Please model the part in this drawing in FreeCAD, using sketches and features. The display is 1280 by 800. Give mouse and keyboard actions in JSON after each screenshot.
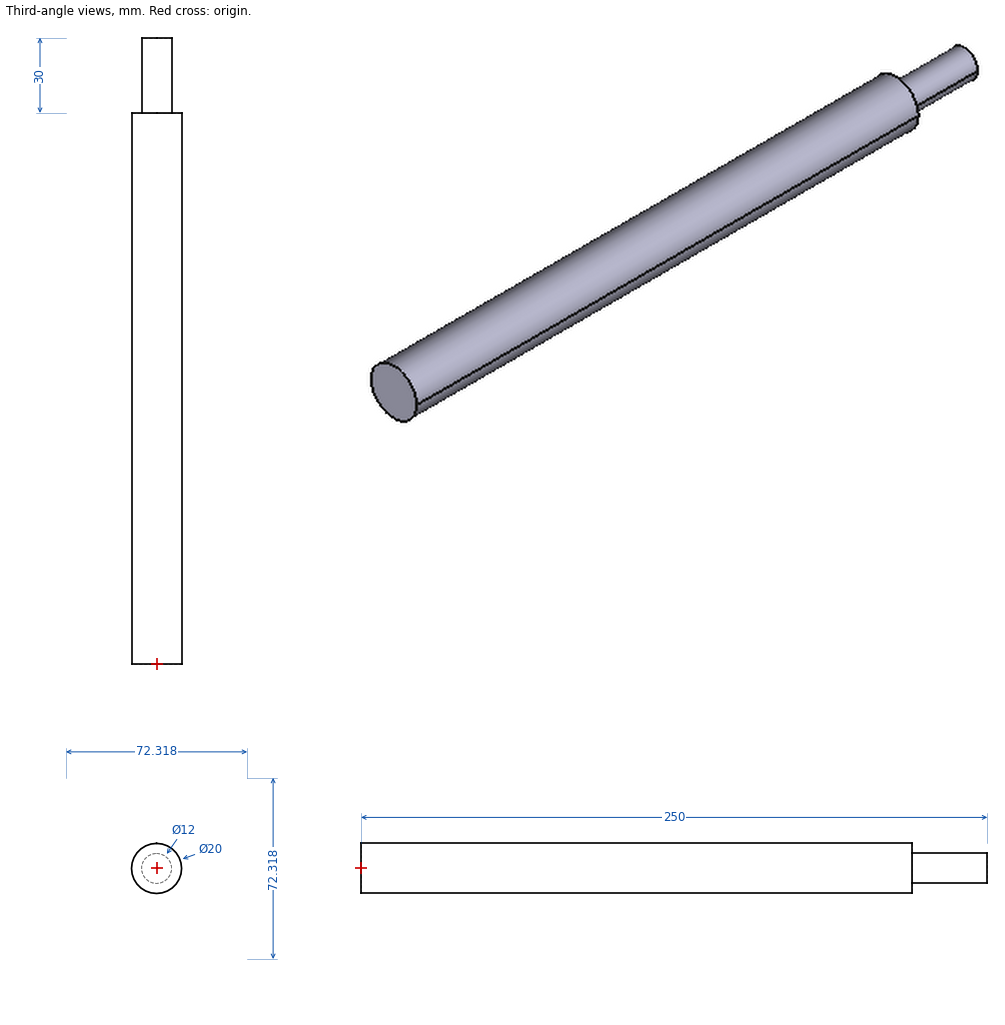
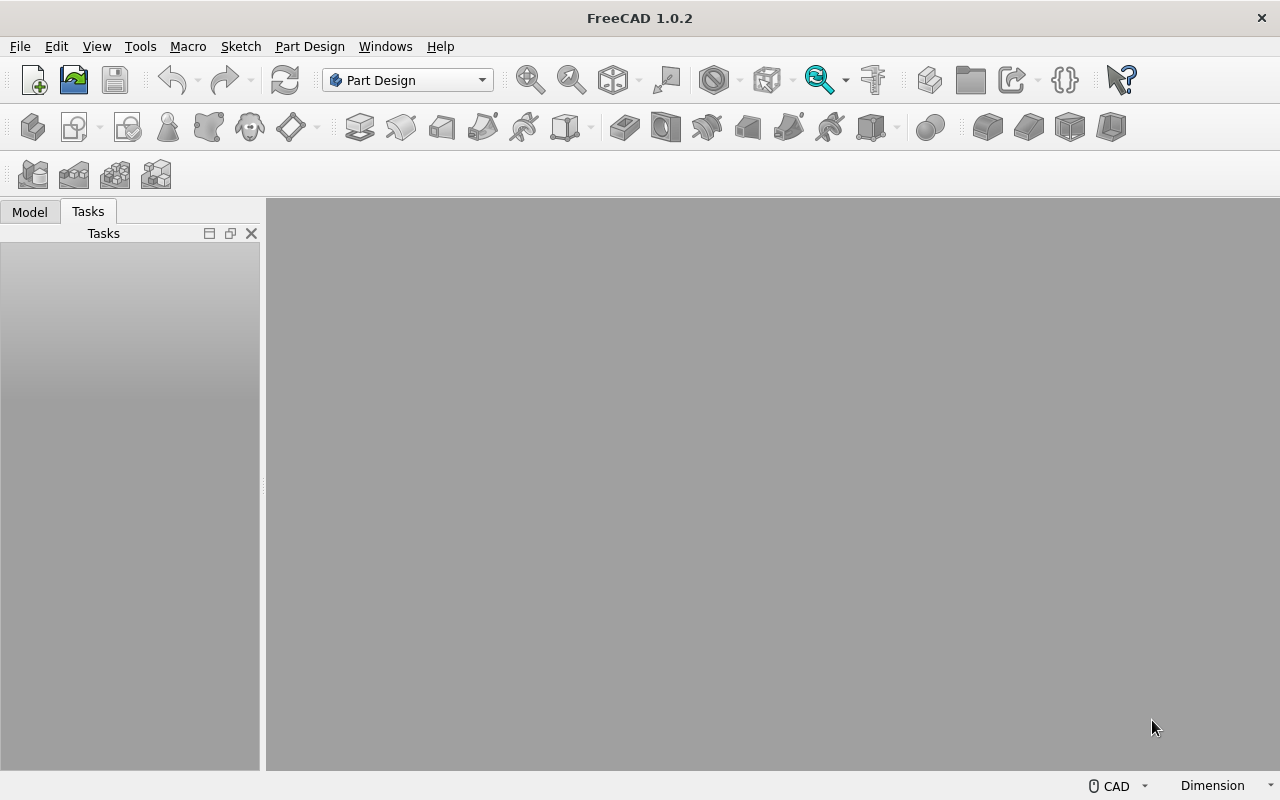
{"action": "left_click", "coordinate": [33, 80]}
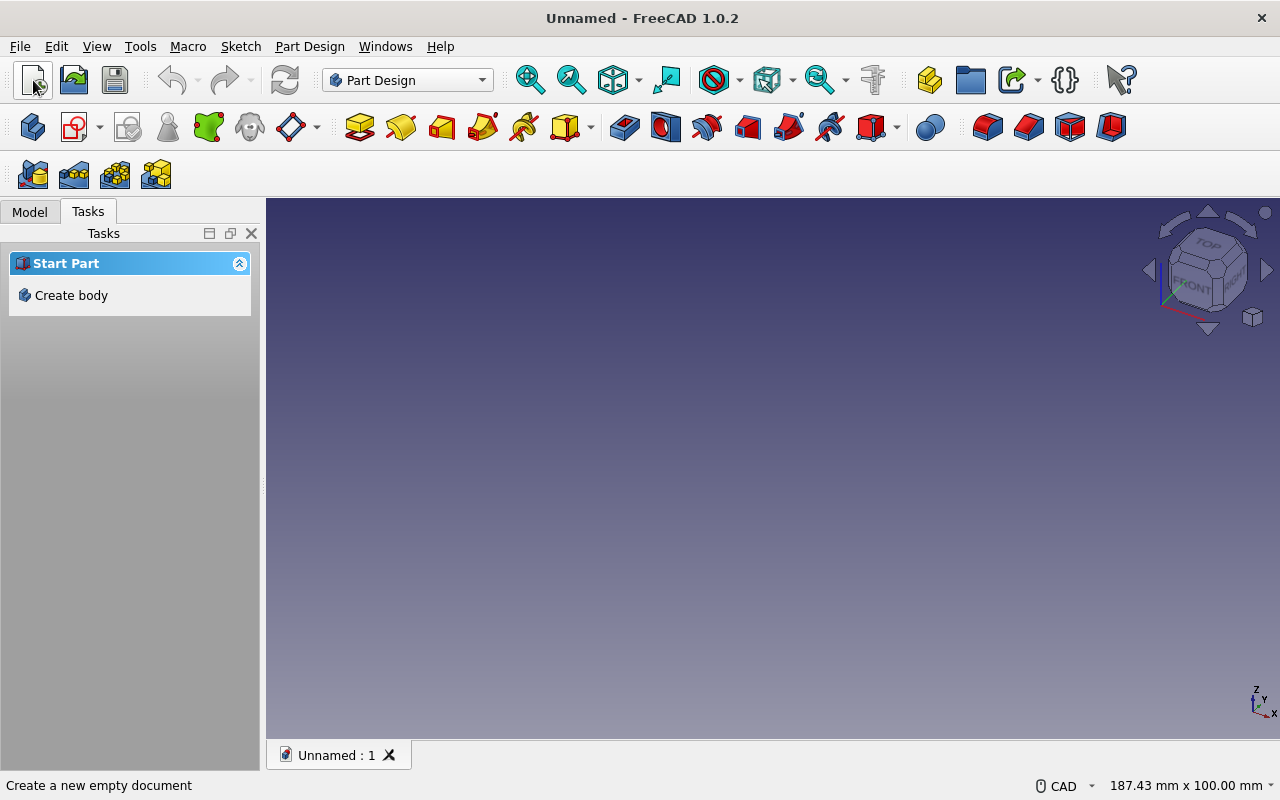
{"action": "left_click", "coordinate": [74, 128]}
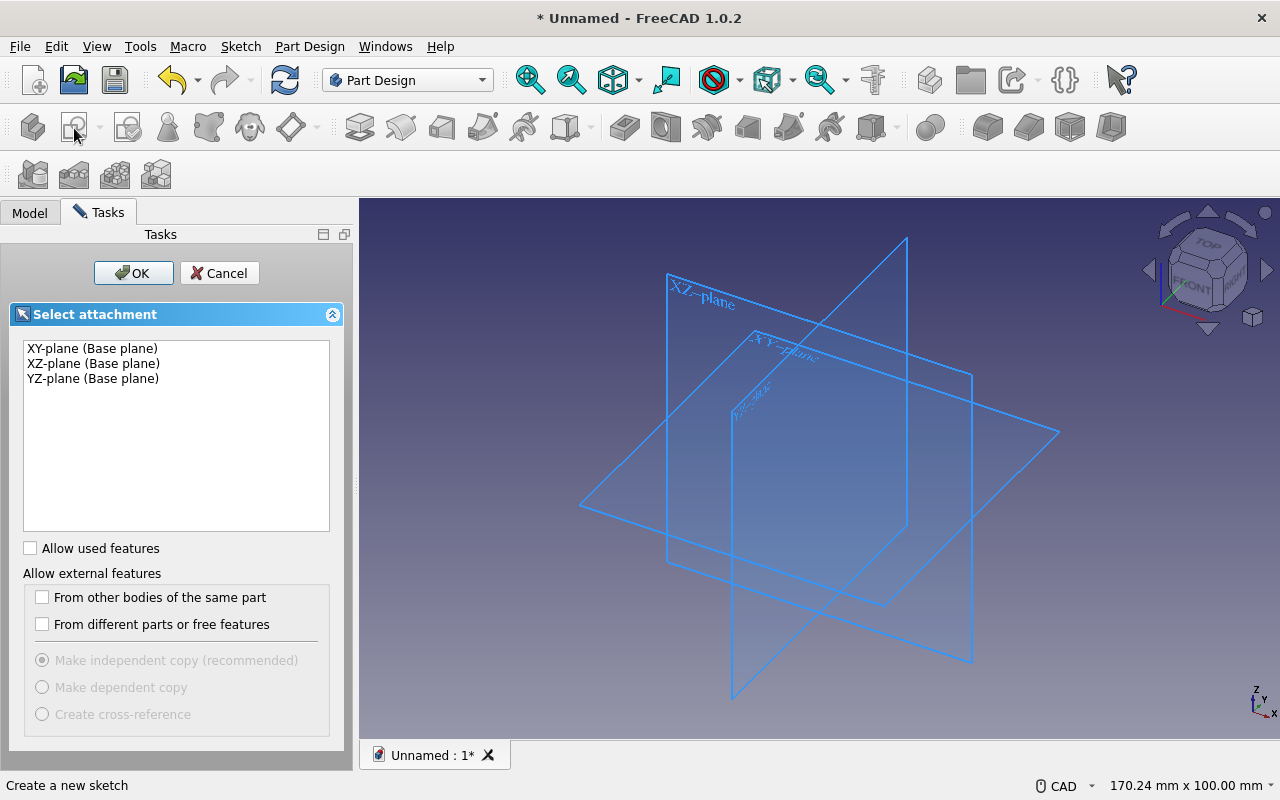
{"action": "left_click", "coordinate": [84, 364]}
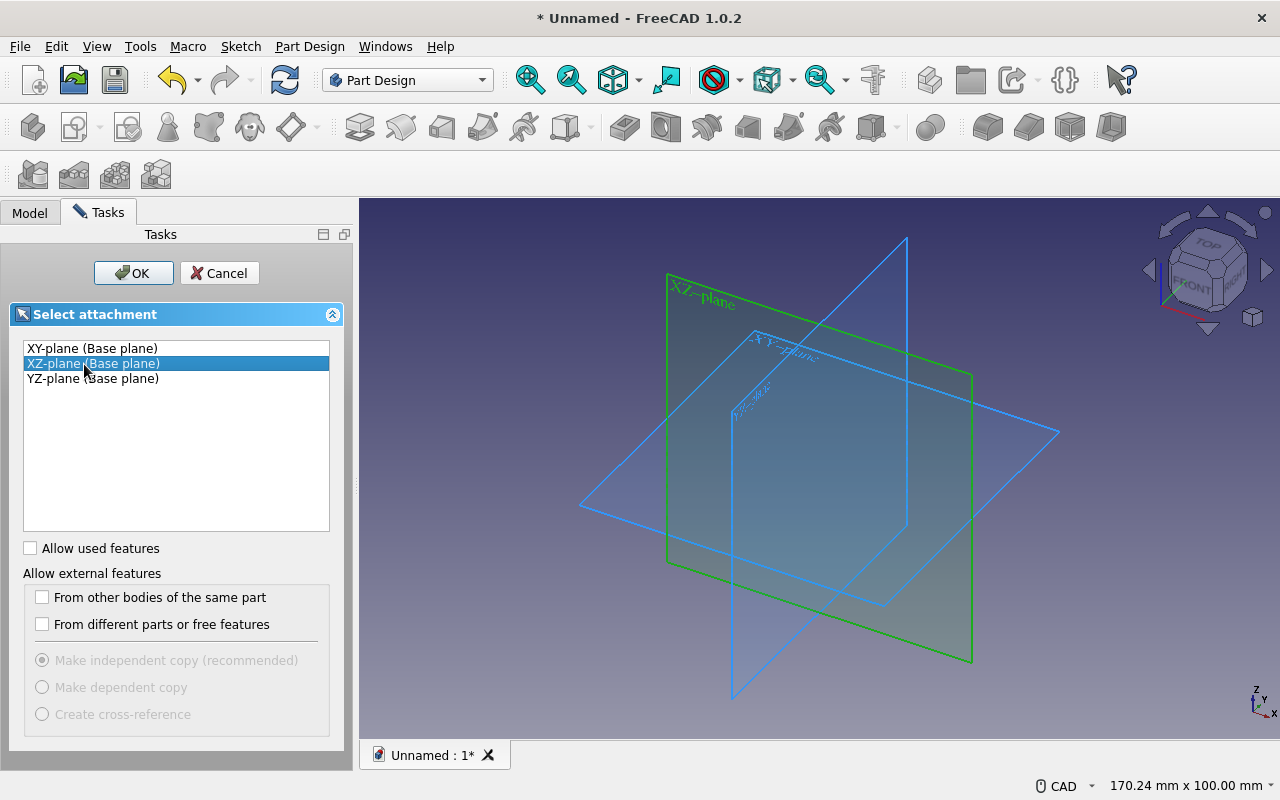
{"action": "left_click", "coordinate": [134, 273]}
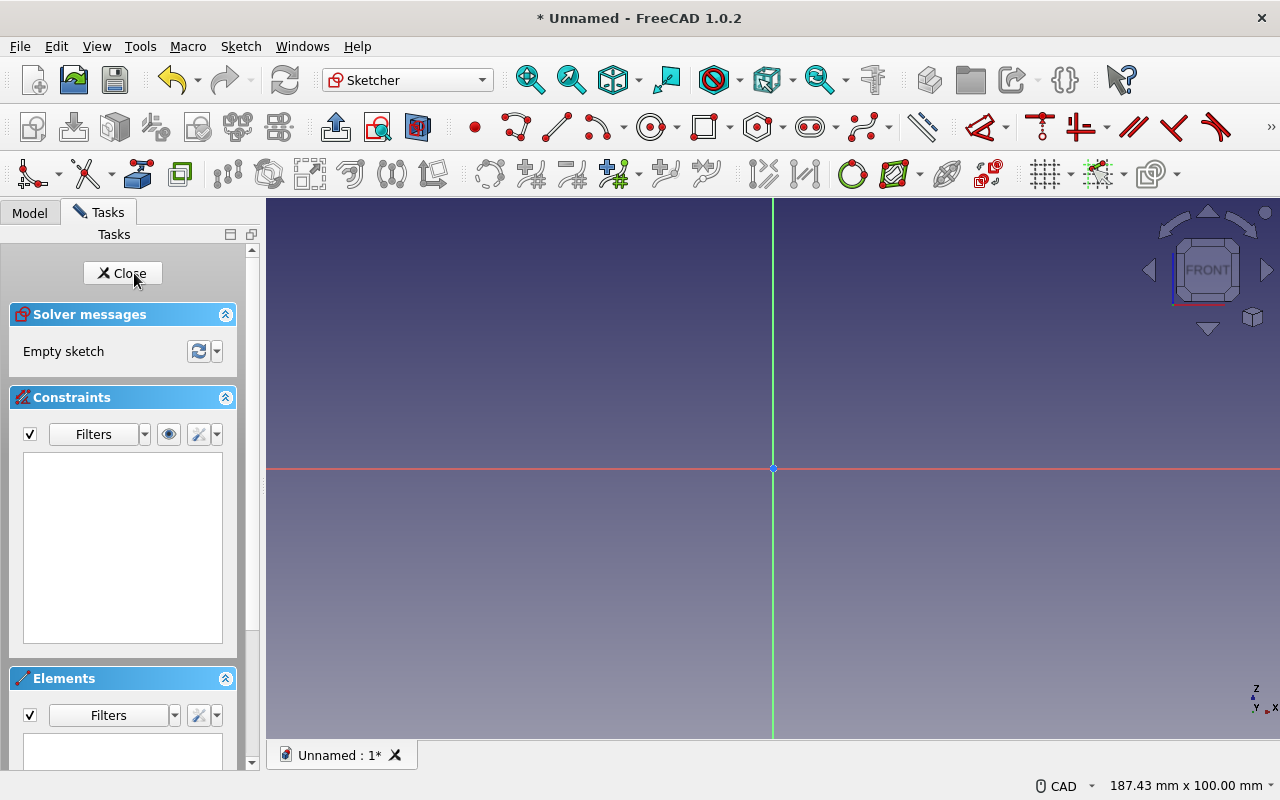
{"action": "scroll", "coordinate": [803, 468], "scroll_direction": "up", "scroll_amount": 6}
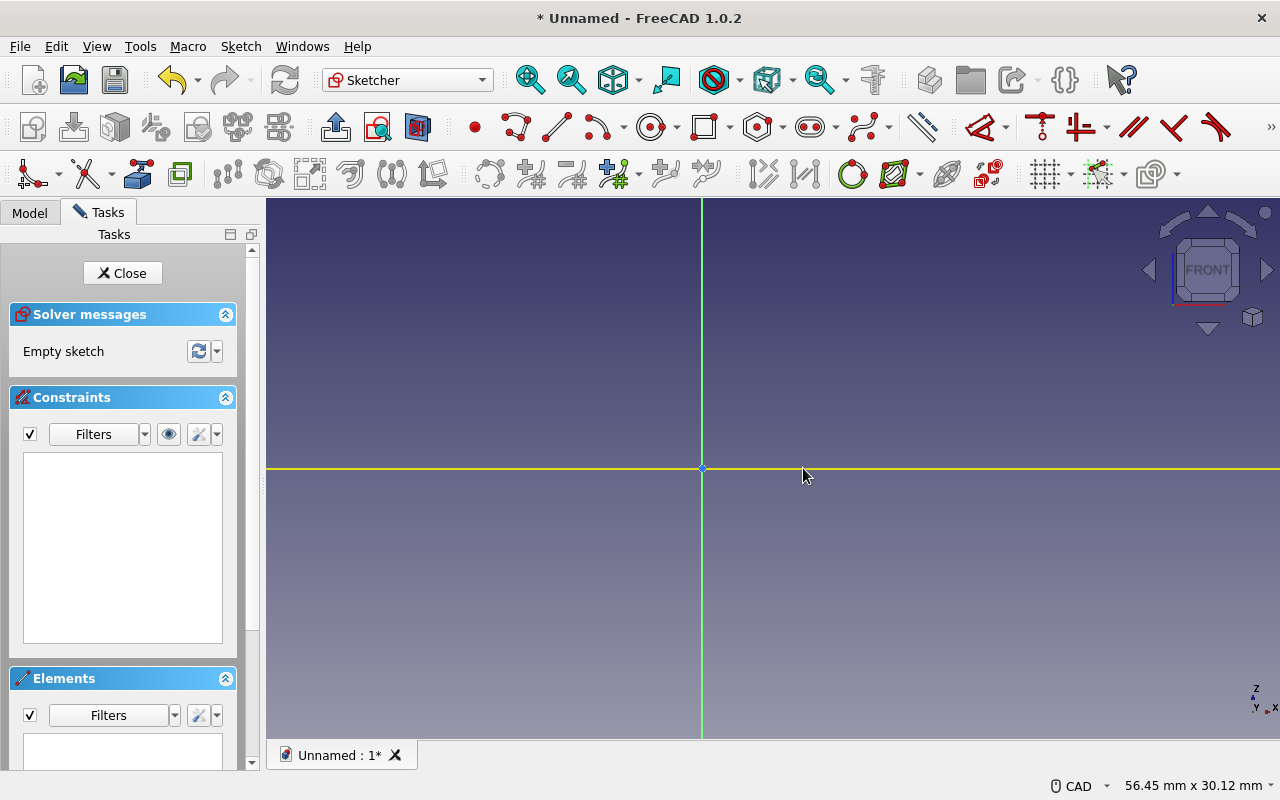
{"action": "left_click", "coordinate": [650, 128]}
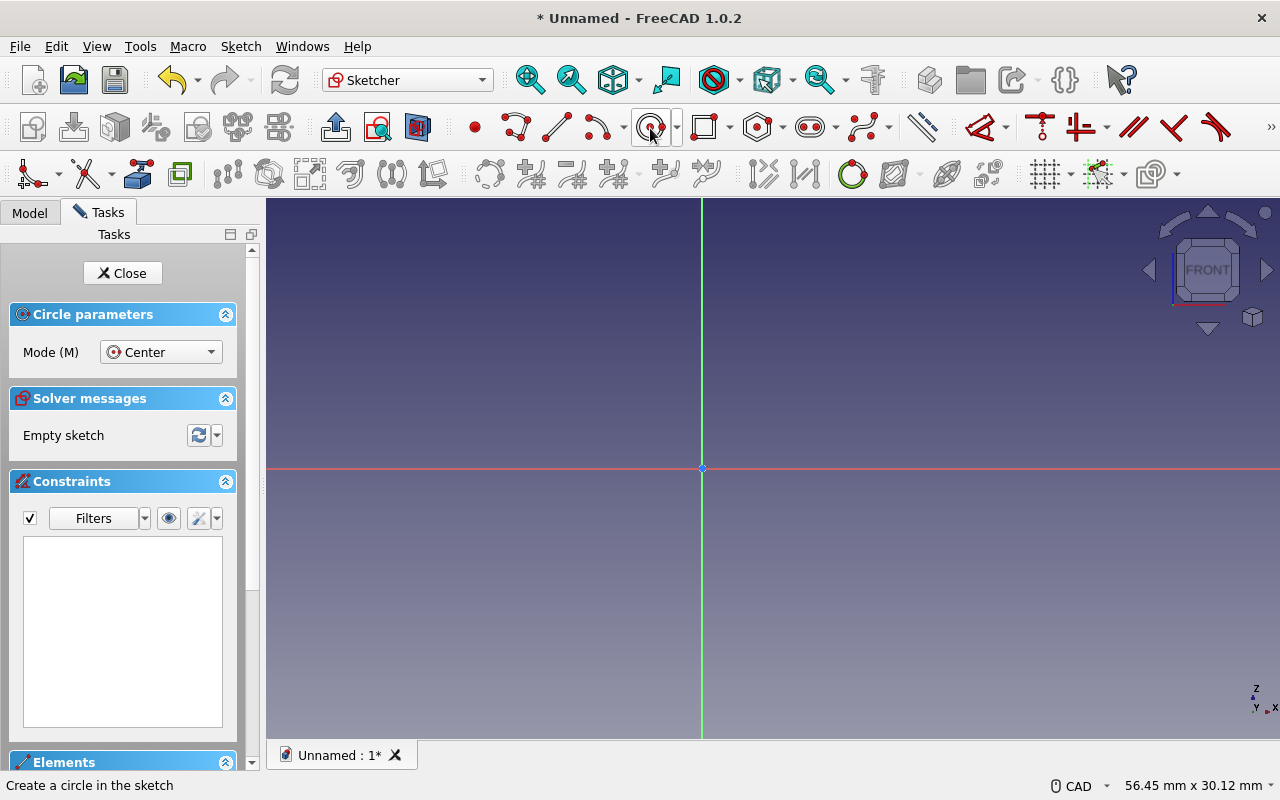
{"action": "left_click", "coordinate": [702, 468]}
{"action": "left_click", "coordinate": [829, 341]}
{"action": "key", "text": "Escape"}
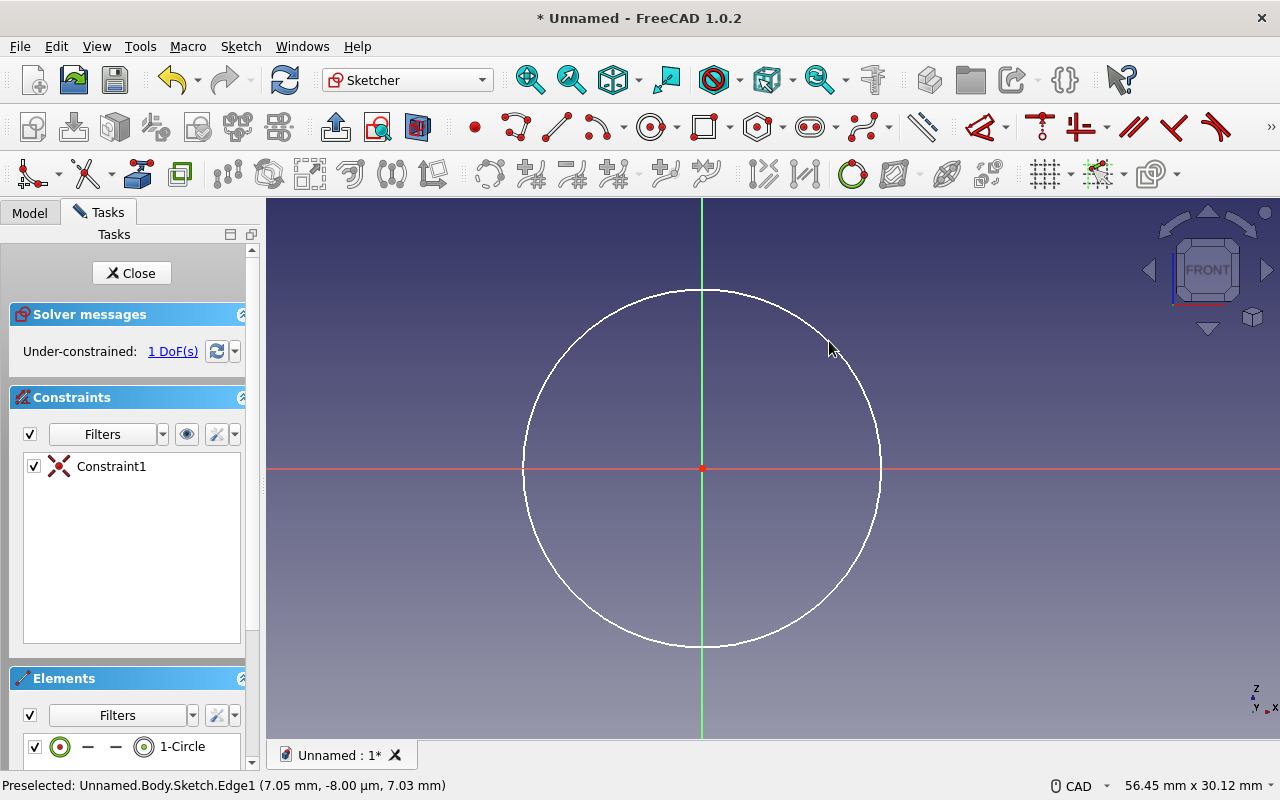
{"action": "key", "text": "d"}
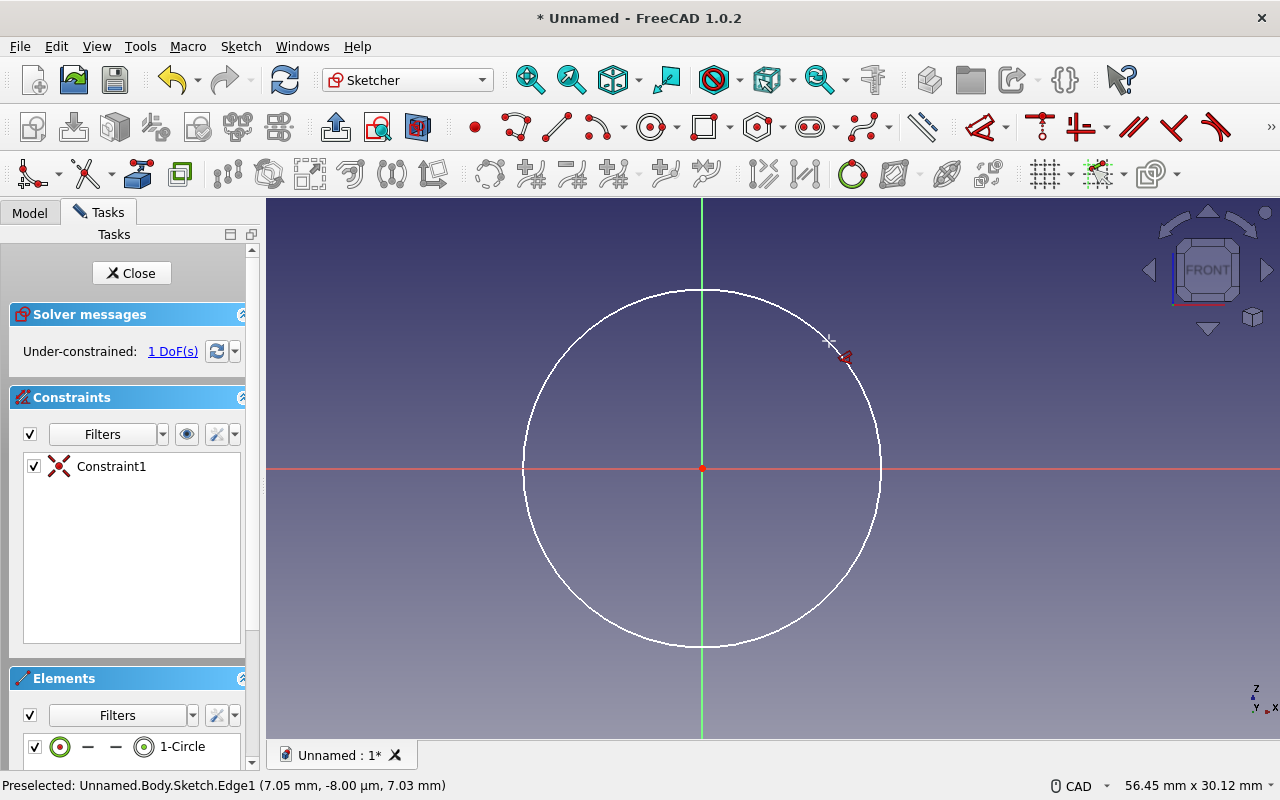
{"action": "left_click", "coordinate": [828, 341]}
{"action": "left_click", "coordinate": [850, 318]}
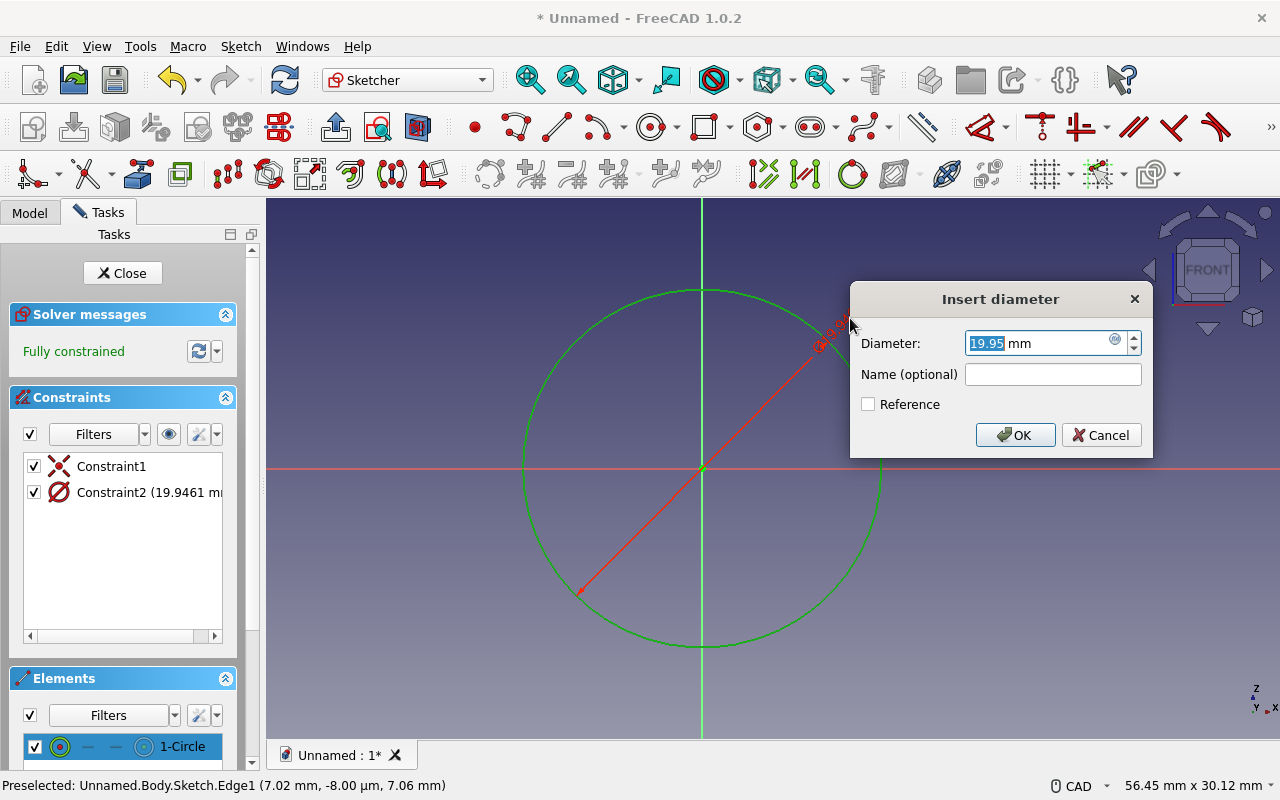
{"action": "type", "text": "20"}
{"action": "key", "text": "Return"}
{"action": "key", "text": "Escape"}